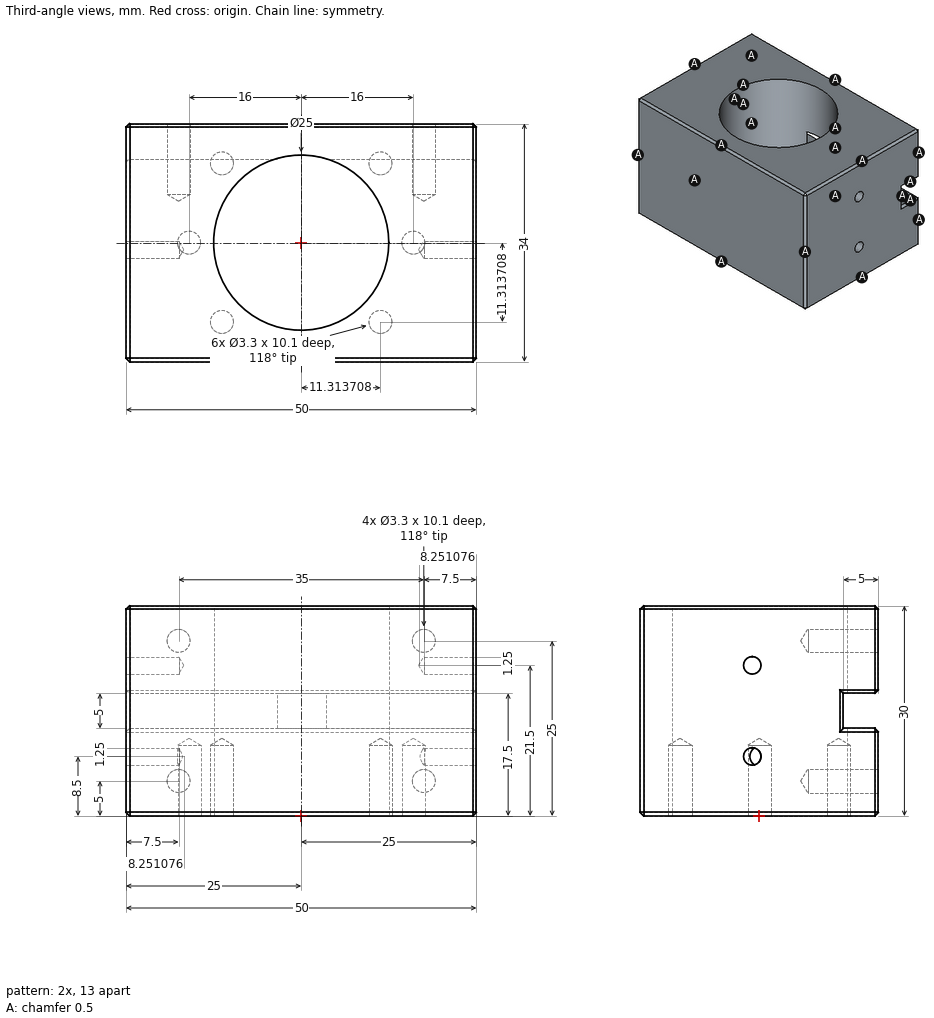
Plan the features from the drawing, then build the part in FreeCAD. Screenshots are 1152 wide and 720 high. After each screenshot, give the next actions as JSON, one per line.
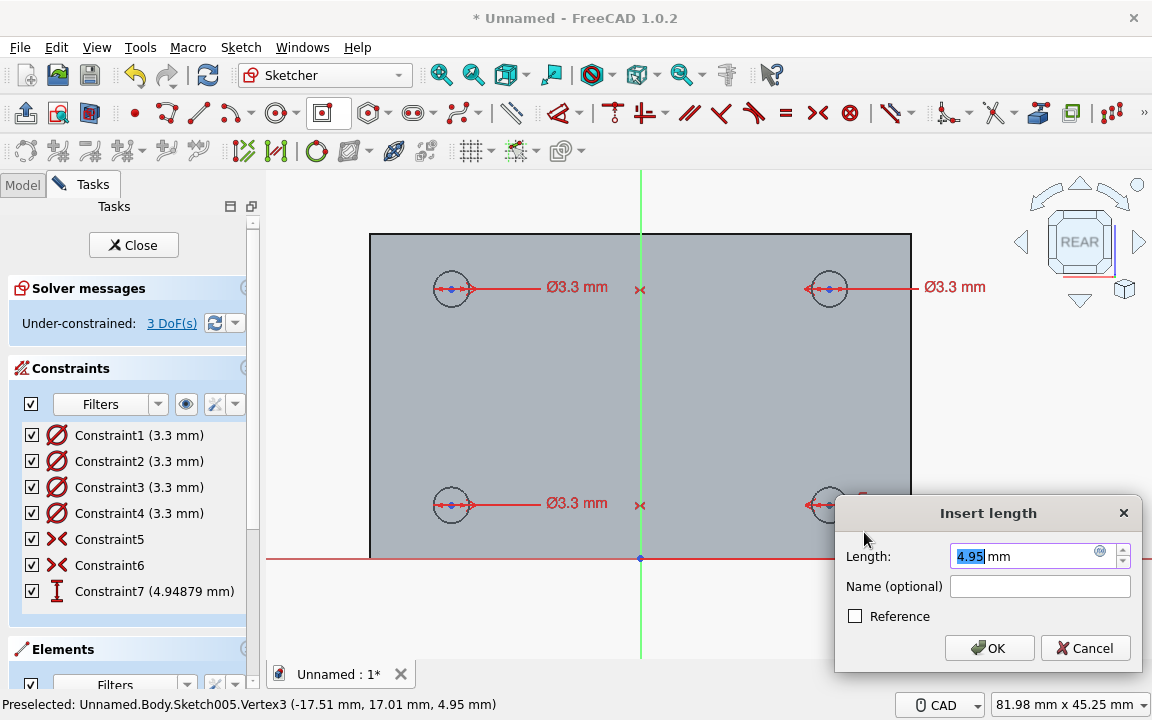
{"action": "type", "text": "5"}
{"action": "key", "text": "Return"}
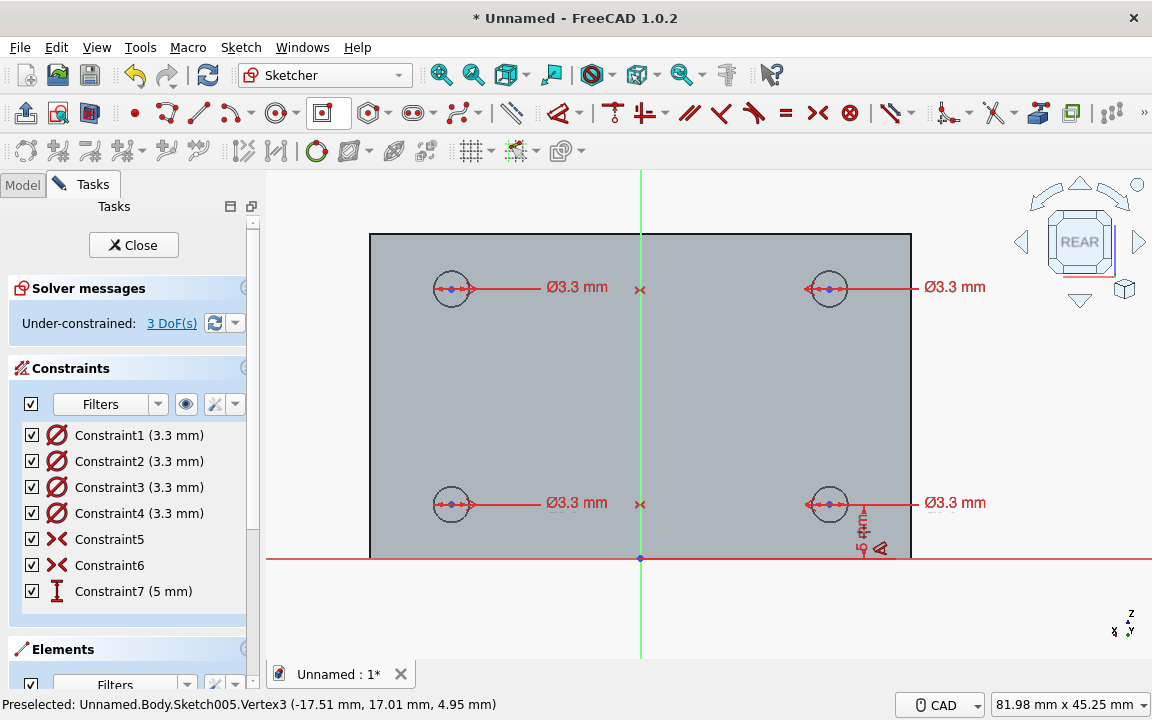
{"action": "left_click", "coordinate": [452, 289]}
{"action": "left_click", "coordinate": [418, 424]}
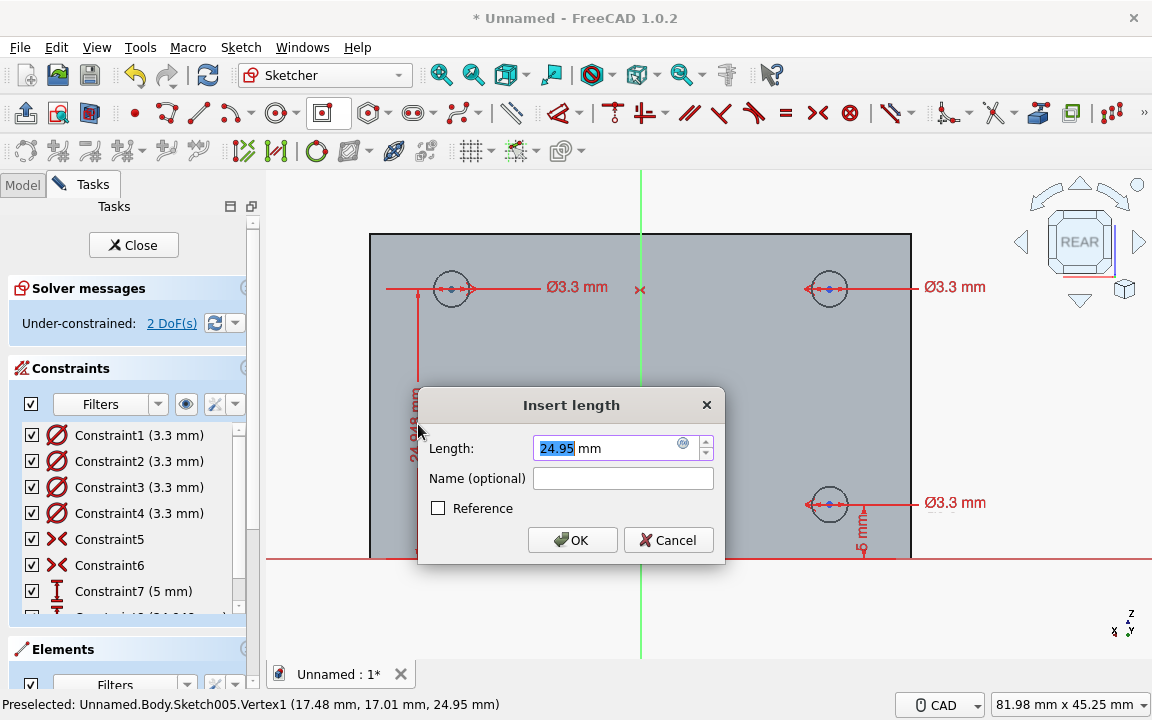
{"action": "type", "text": "25"}
{"action": "key", "text": "Return"}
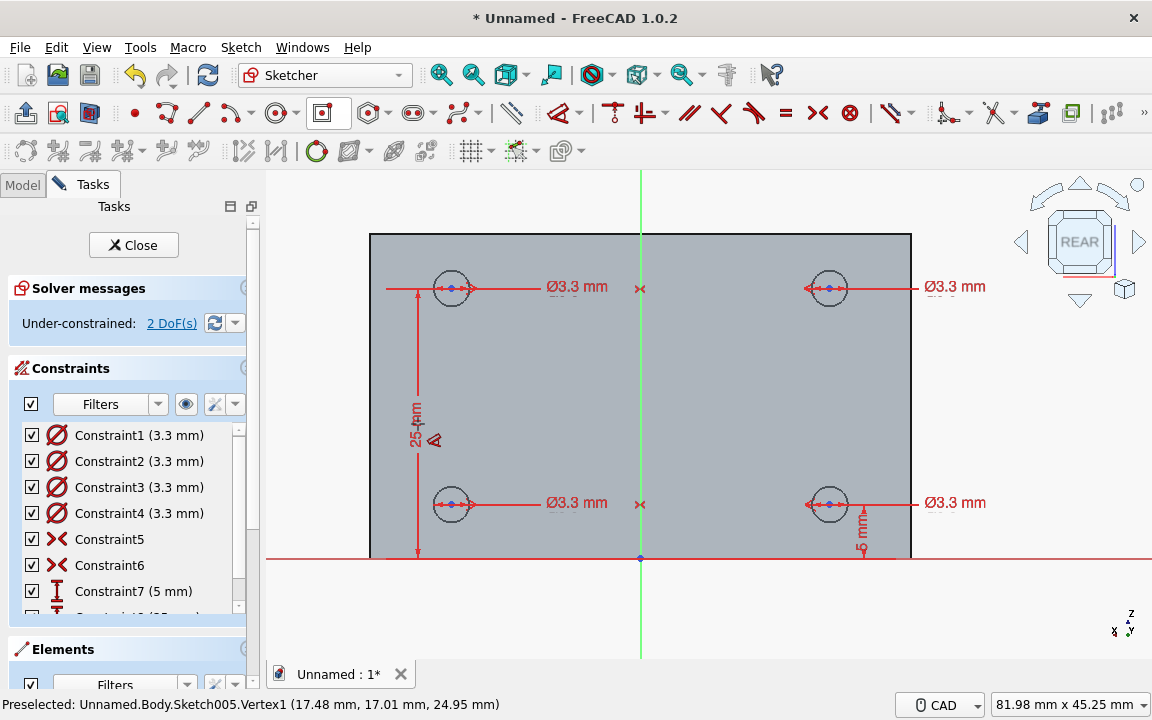
{"action": "left_click", "coordinate": [452, 289]}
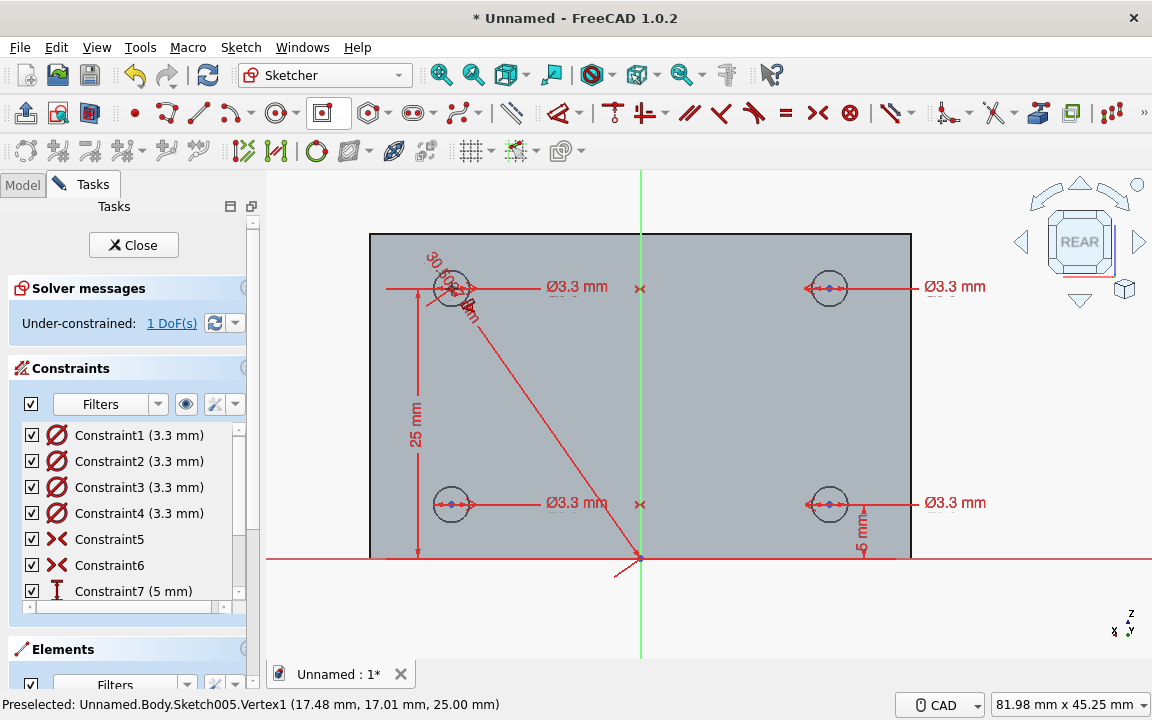
{"action": "left_click", "coordinate": [830, 289]}
{"action": "left_click", "coordinate": [554, 255]}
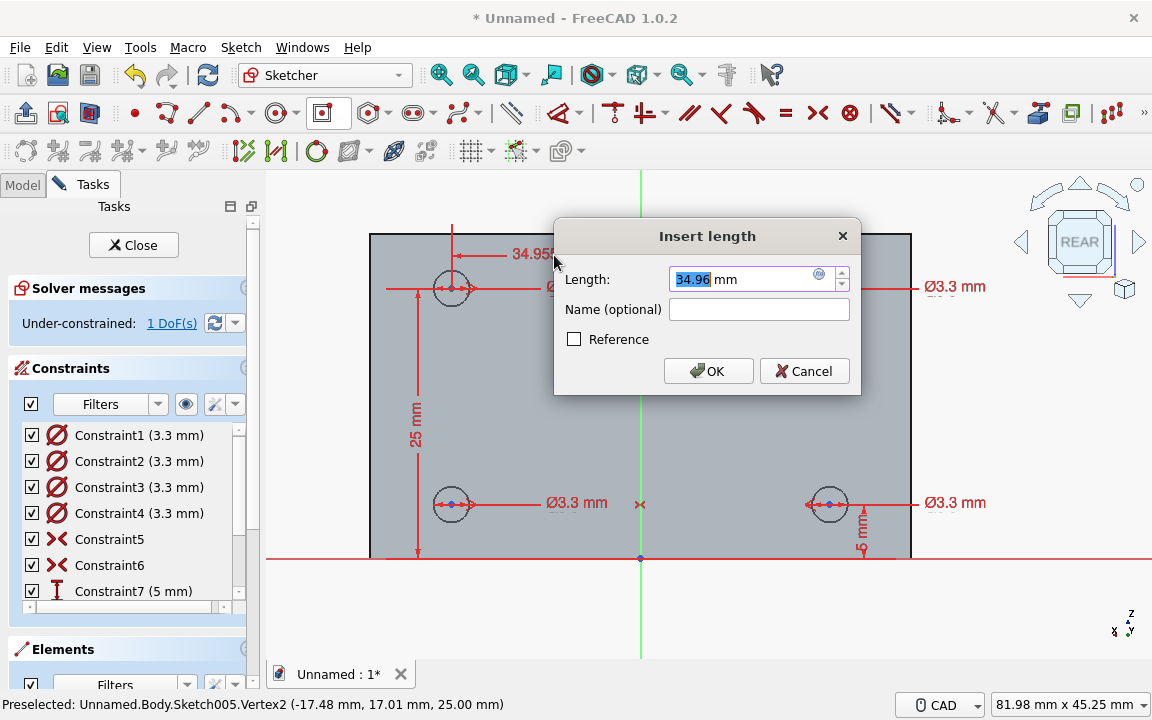
{"action": "type", "text": "35"}
{"action": "key", "text": "Return"}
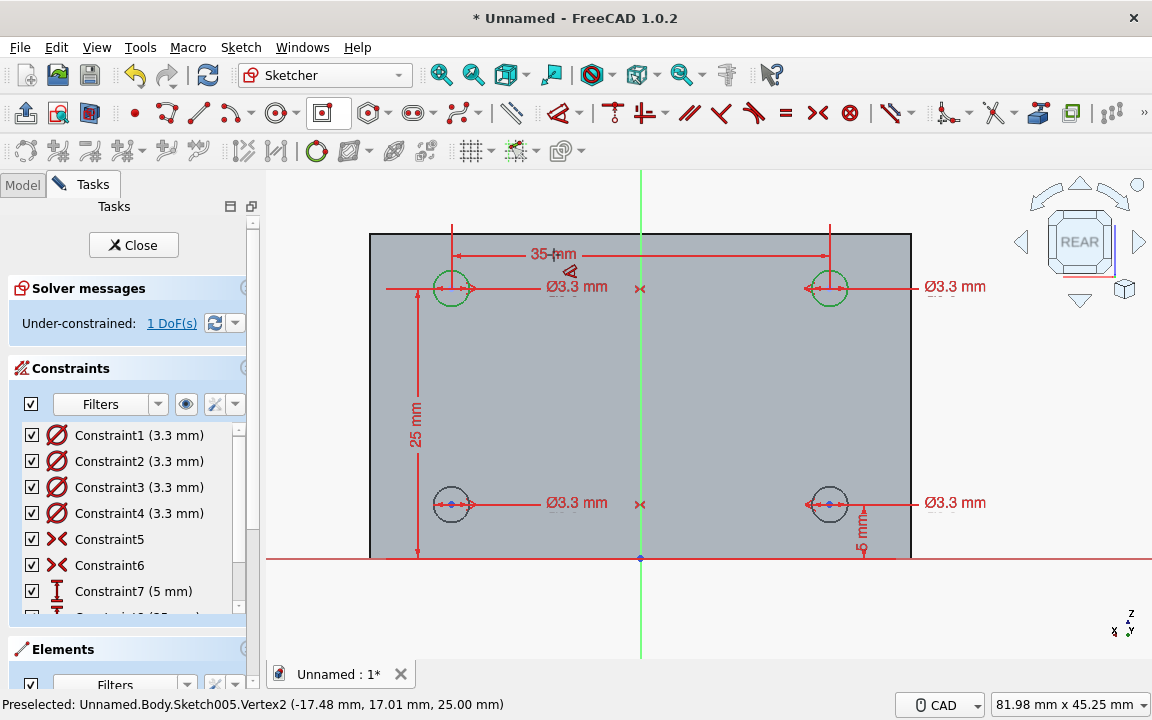
{"action": "left_click", "coordinate": [452, 289]}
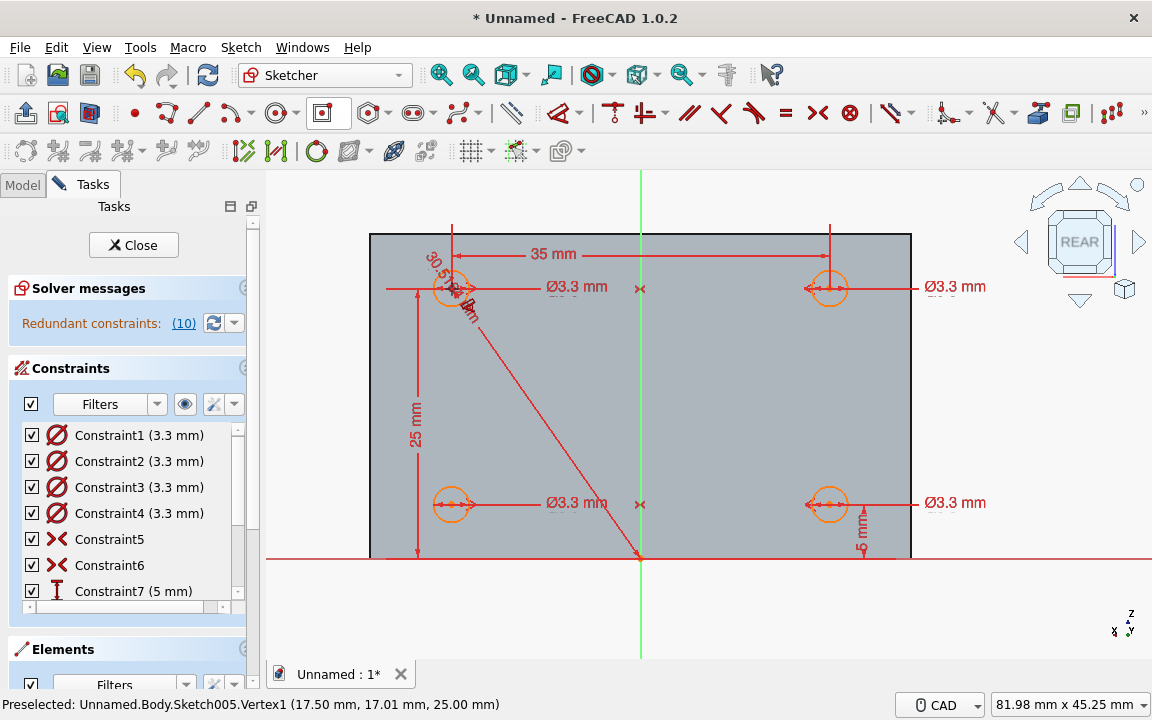
{"action": "left_click", "coordinate": [830, 505]}
{"action": "left_click", "coordinate": [728, 255]}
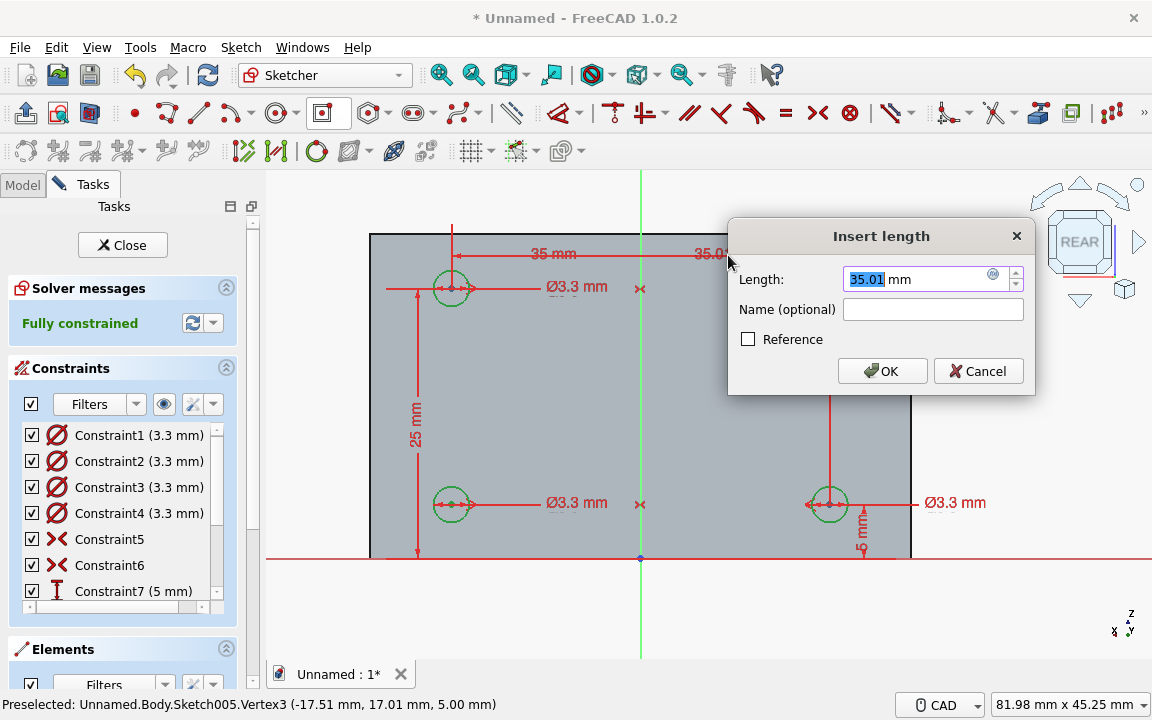
{"action": "type", "text": "35"}
{"action": "key", "text": "Return"}
{"action": "key", "text": "Escape"}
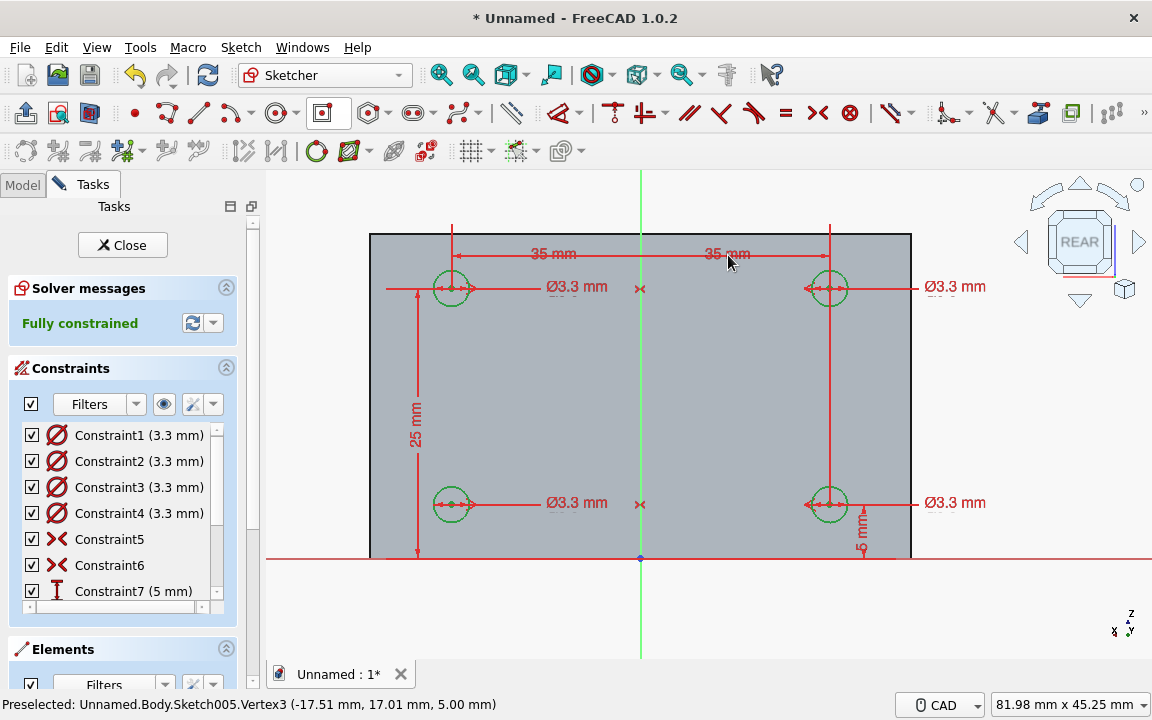
{"action": "left_click", "coordinate": [123, 245]}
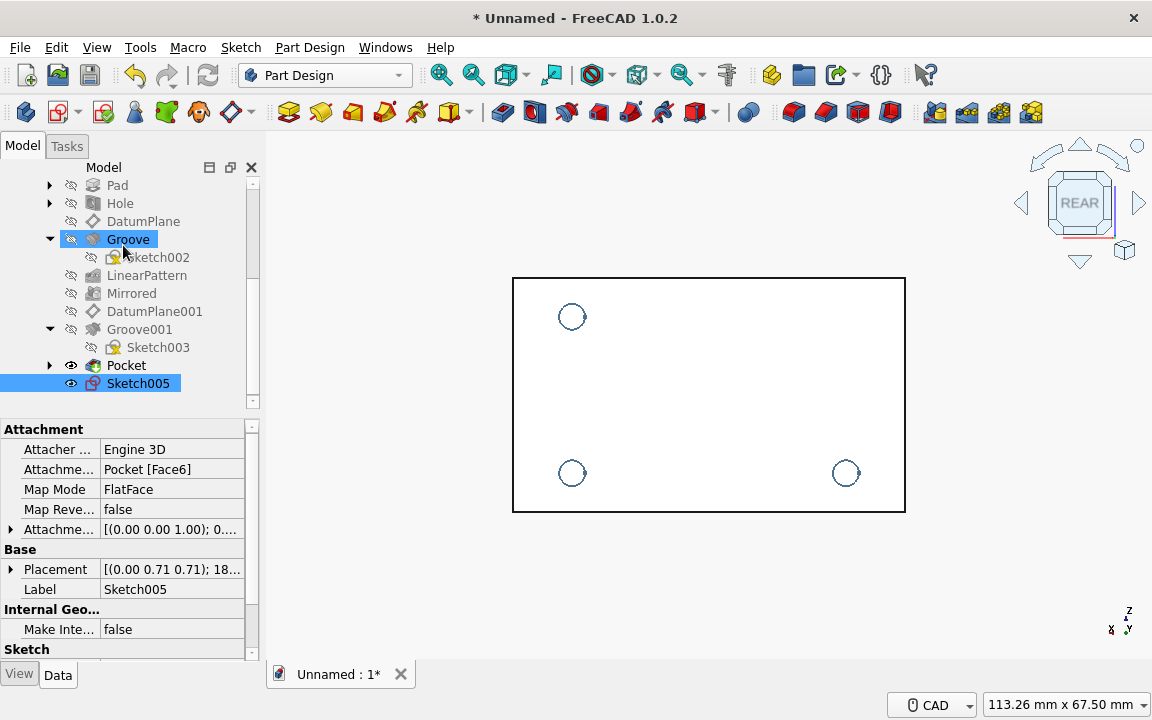
{"action": "left_click", "coordinate": [536, 112]}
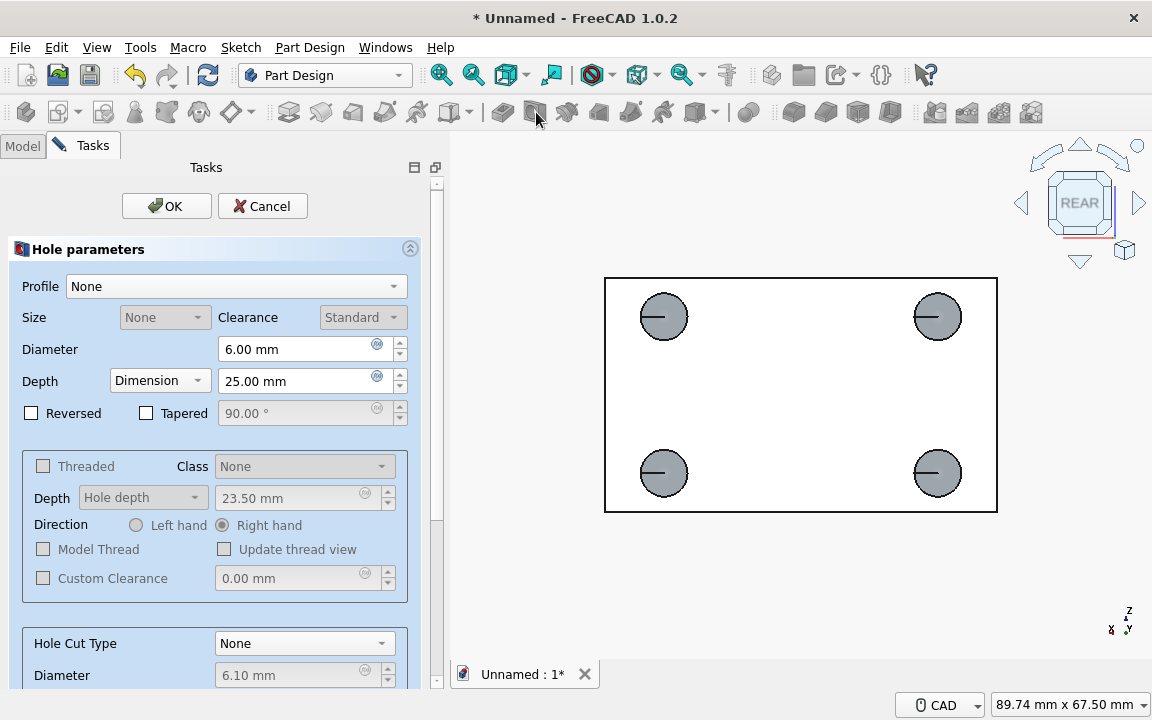
{"action": "triple_click", "coordinate": [305, 349]}